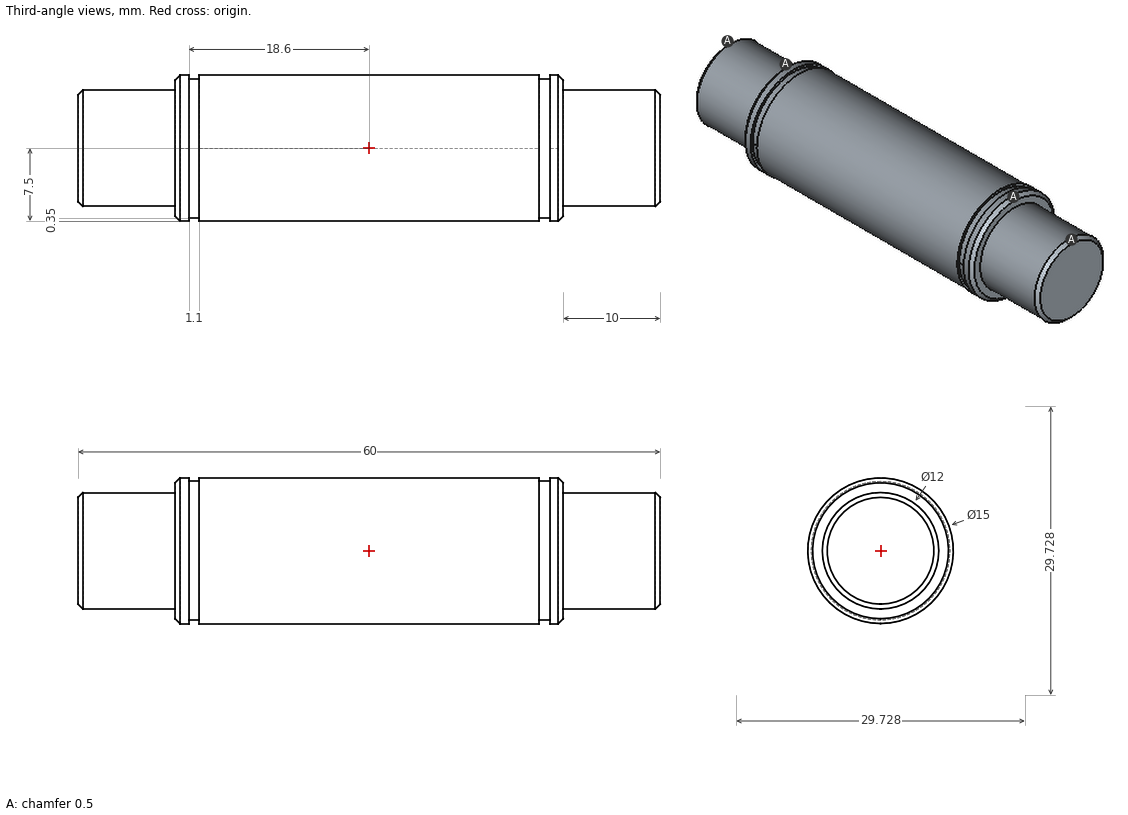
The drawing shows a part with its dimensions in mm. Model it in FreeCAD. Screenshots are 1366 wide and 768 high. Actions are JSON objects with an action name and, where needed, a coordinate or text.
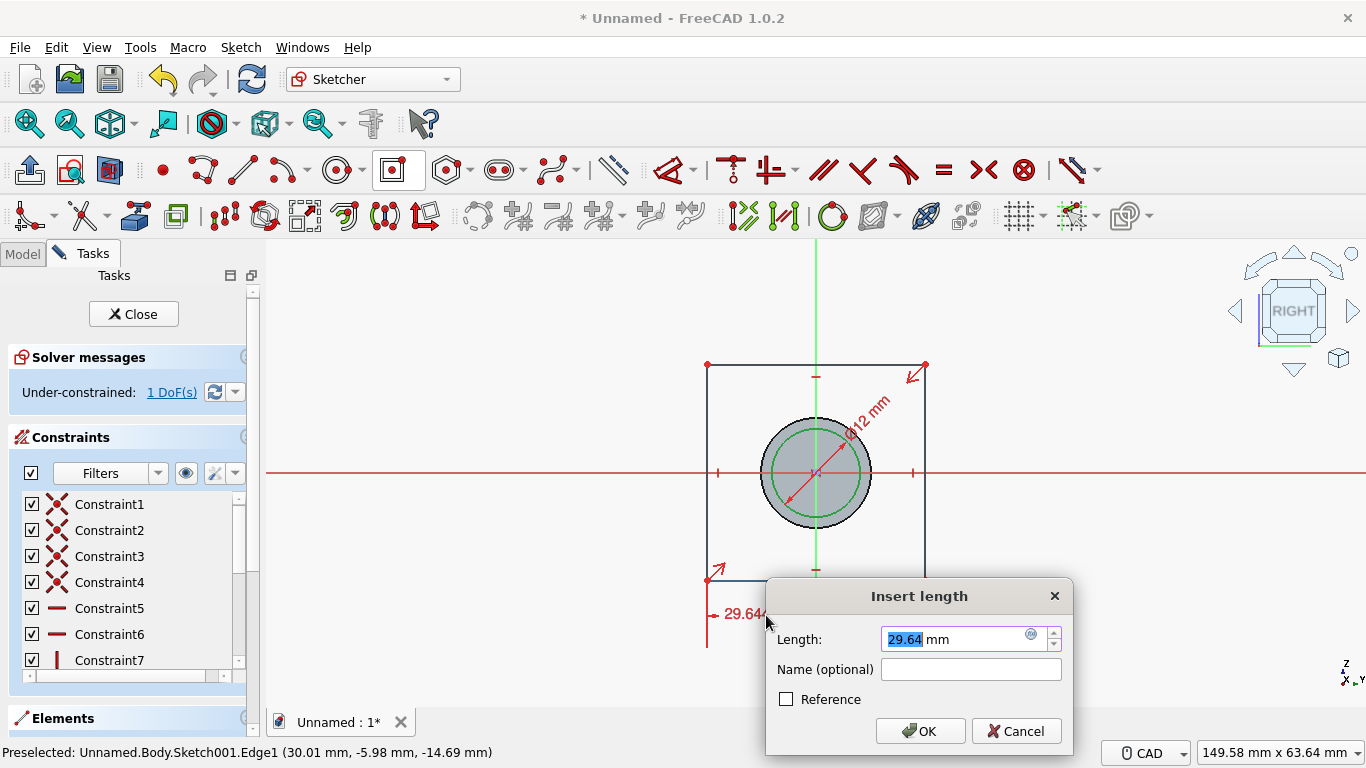
{"action": "type", "text": "29.728"}
{"action": "key", "text": "Return"}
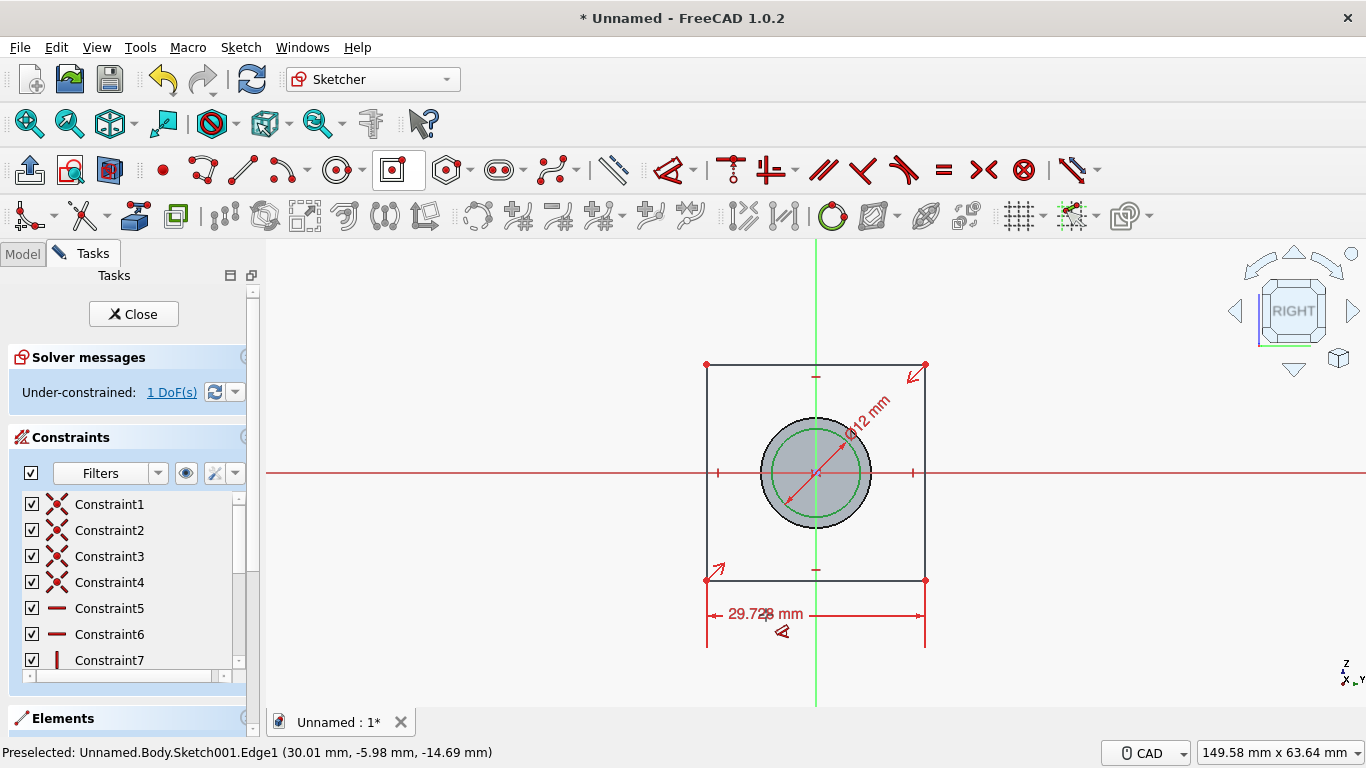
{"action": "left_click", "coordinate": [925, 516]}
{"action": "left_click", "coordinate": [959, 423]}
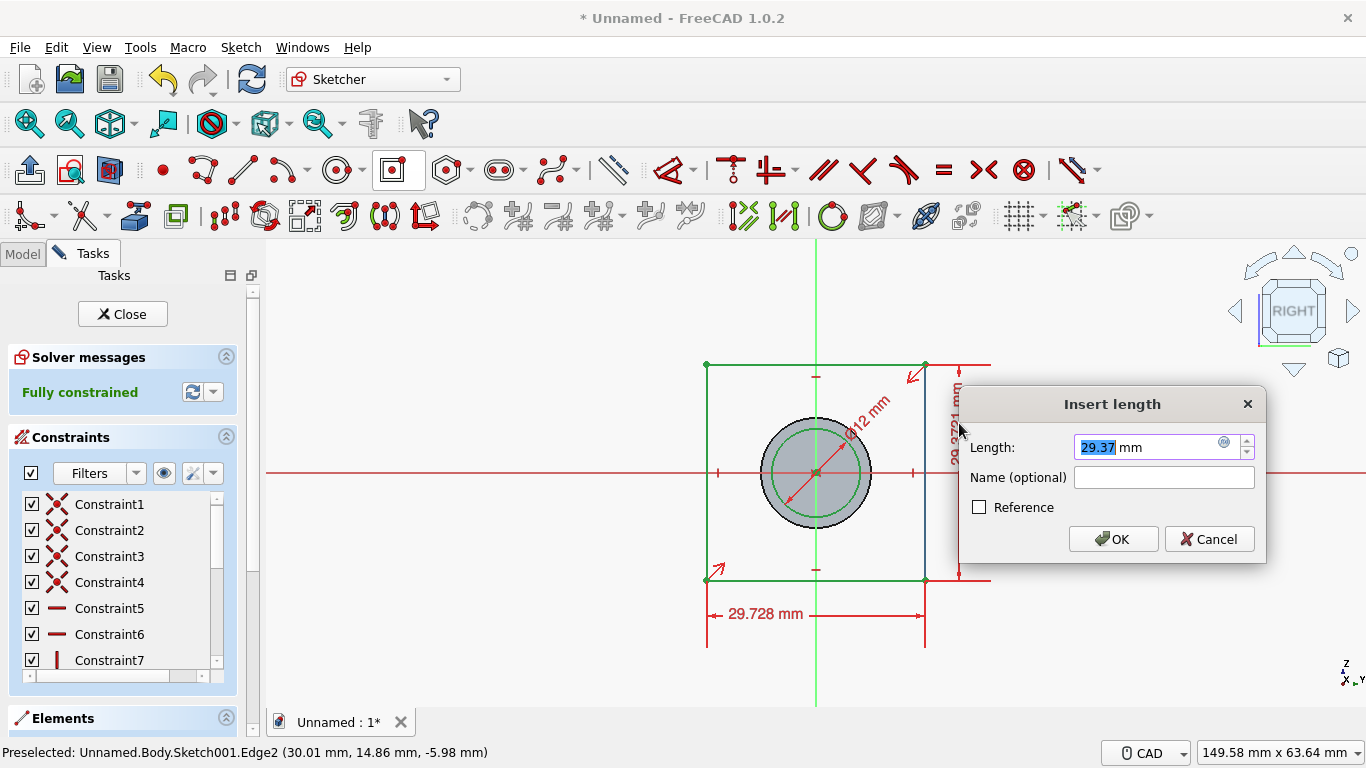
{"action": "type", "text": "29.728"}
{"action": "key", "text": "Return"}
{"action": "key", "text": "Escape"}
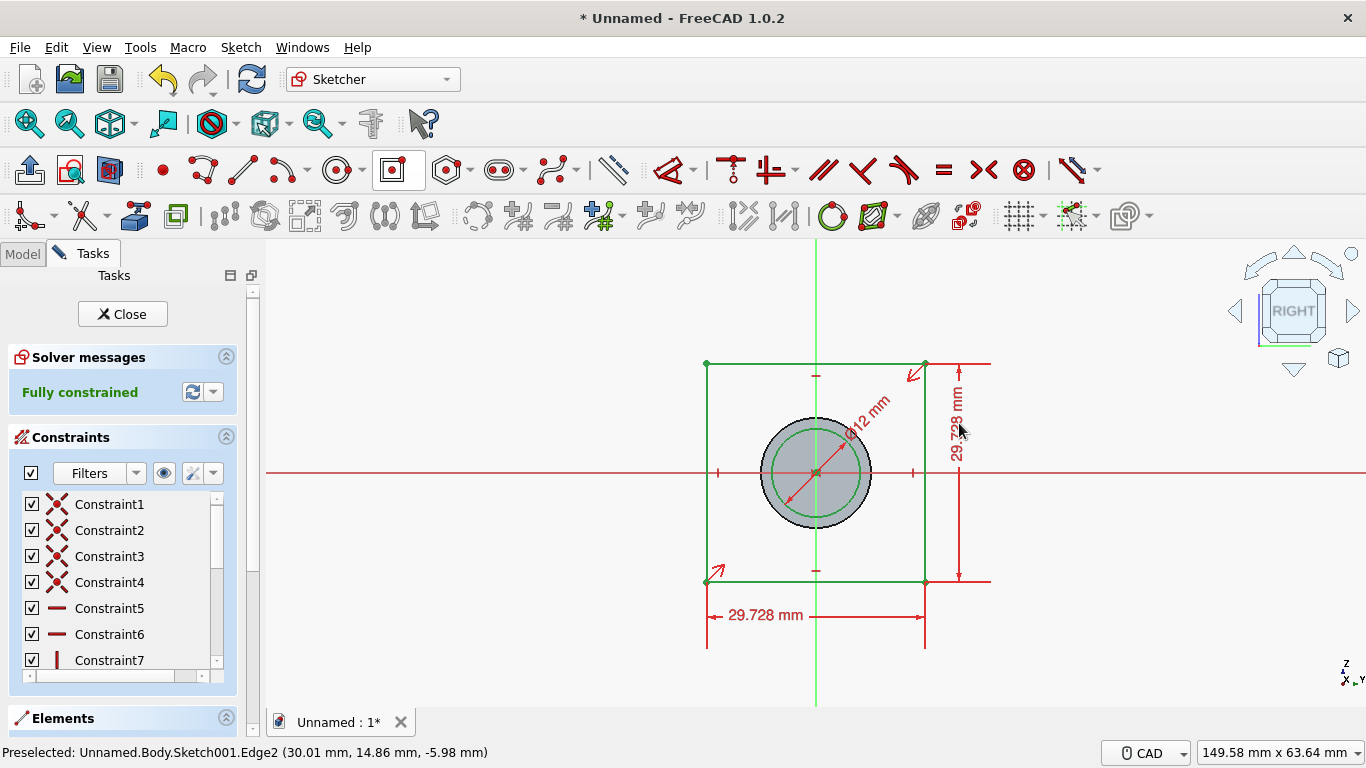
{"action": "left_click", "coordinate": [123, 314]}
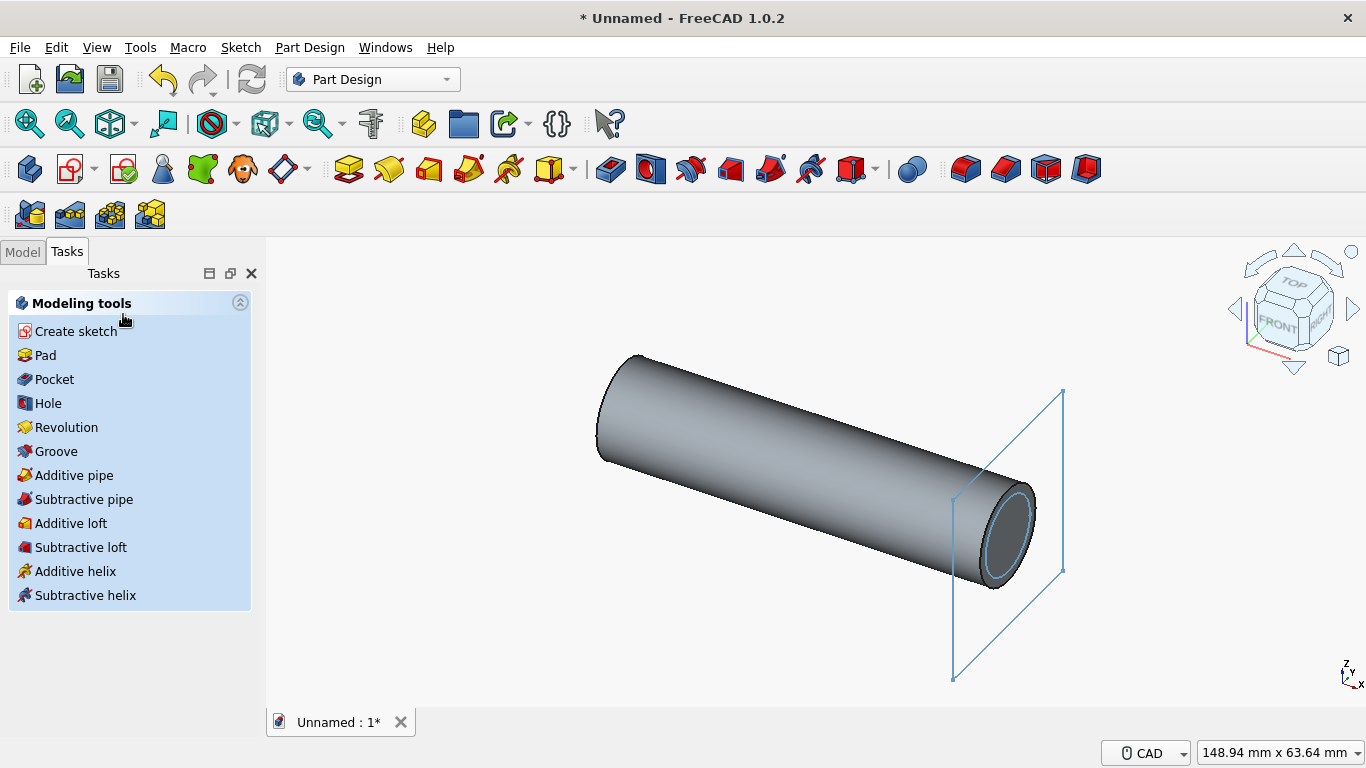
{"action": "left_click", "coordinate": [612, 170]}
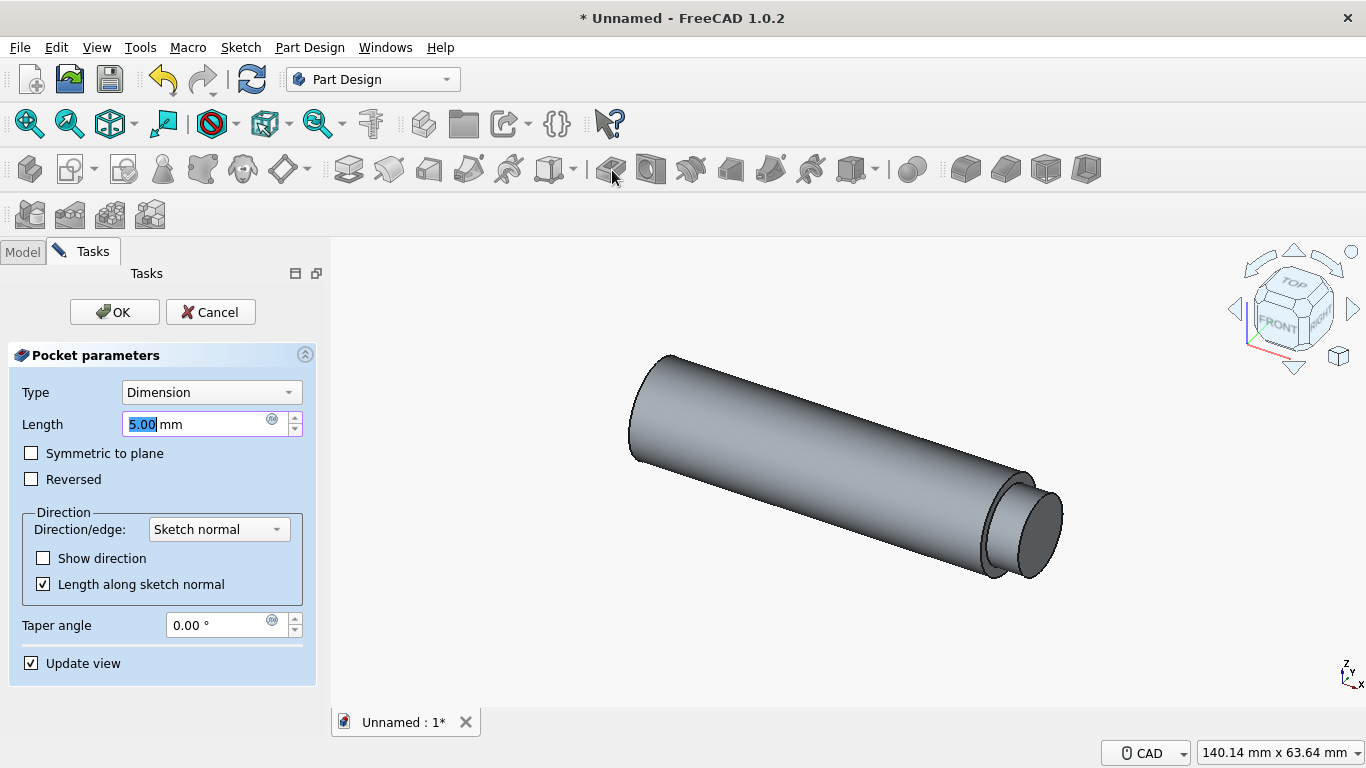
{"action": "type", "text": "10"}
{"action": "key", "text": "Tab"}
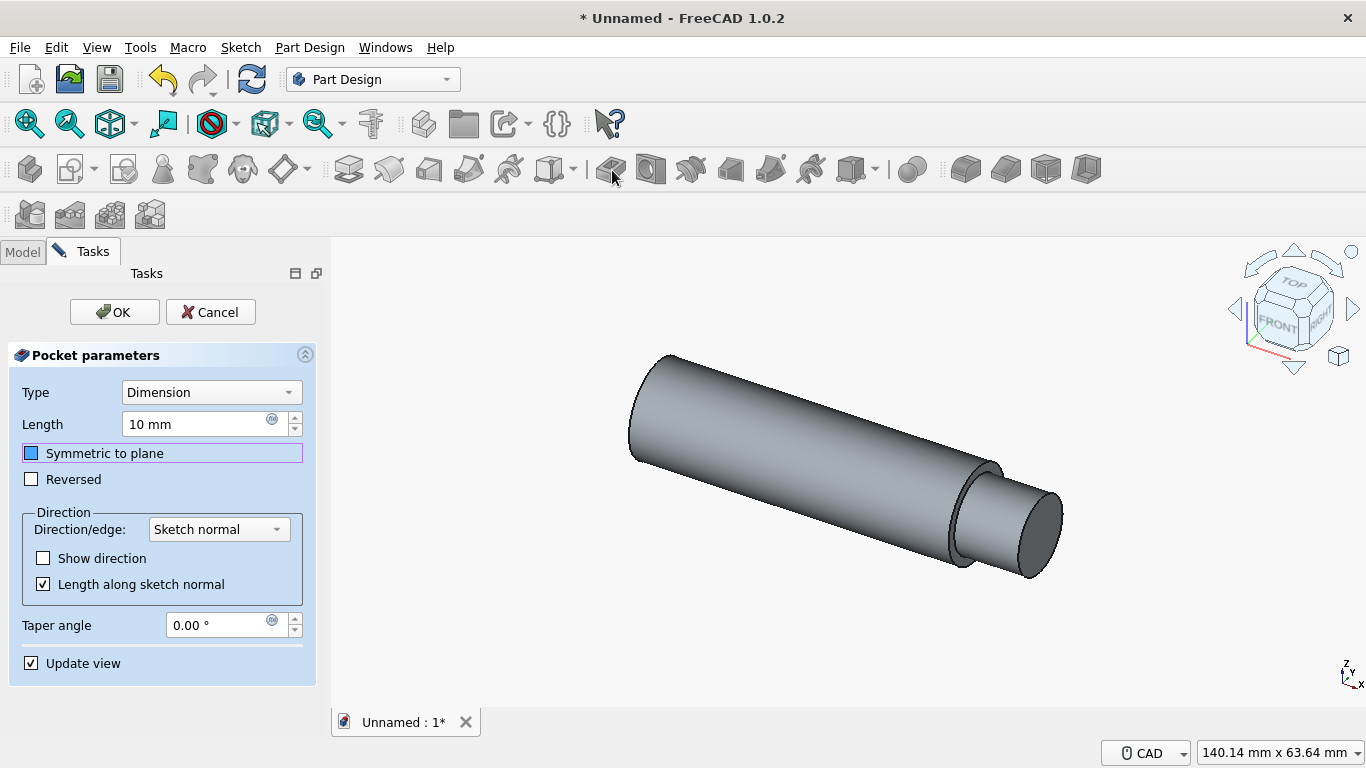
{"action": "left_click", "coordinate": [115, 312]}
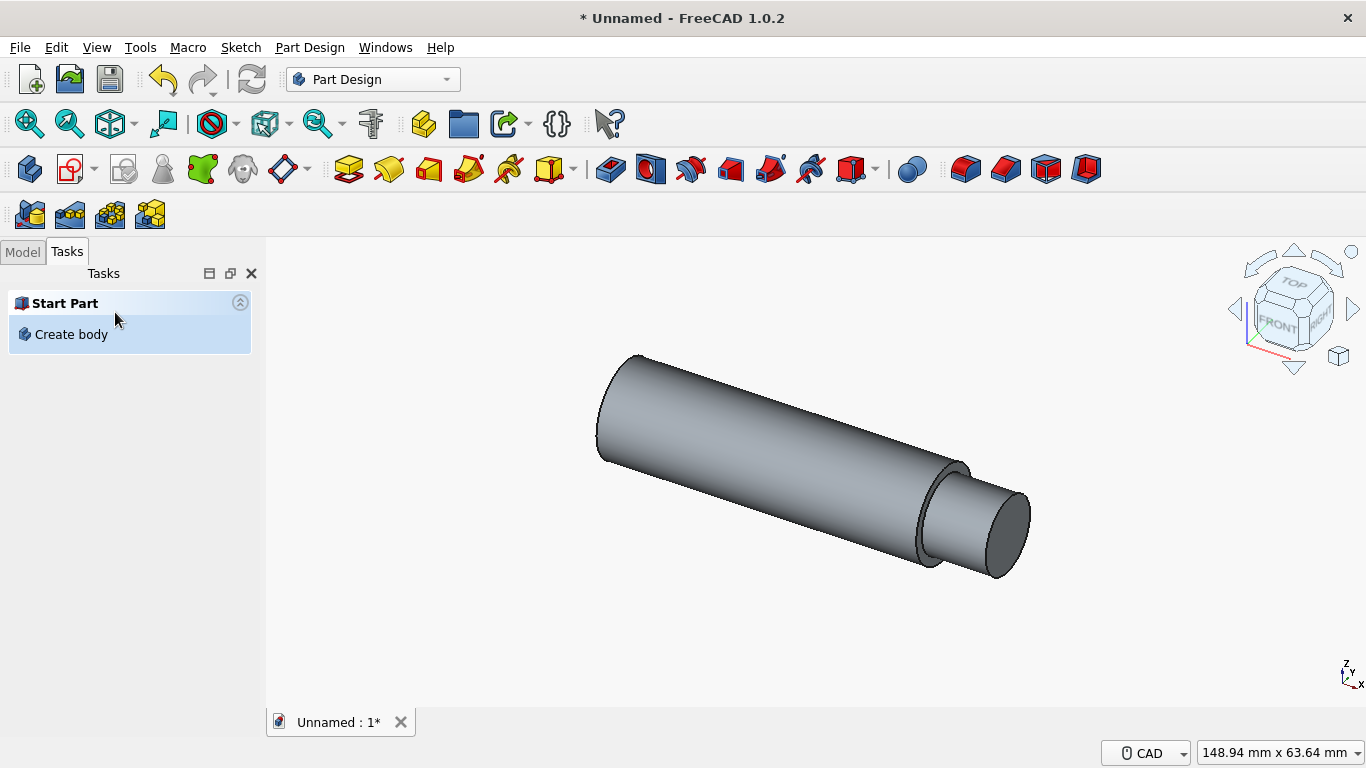
{"action": "left_click", "coordinate": [23, 251]}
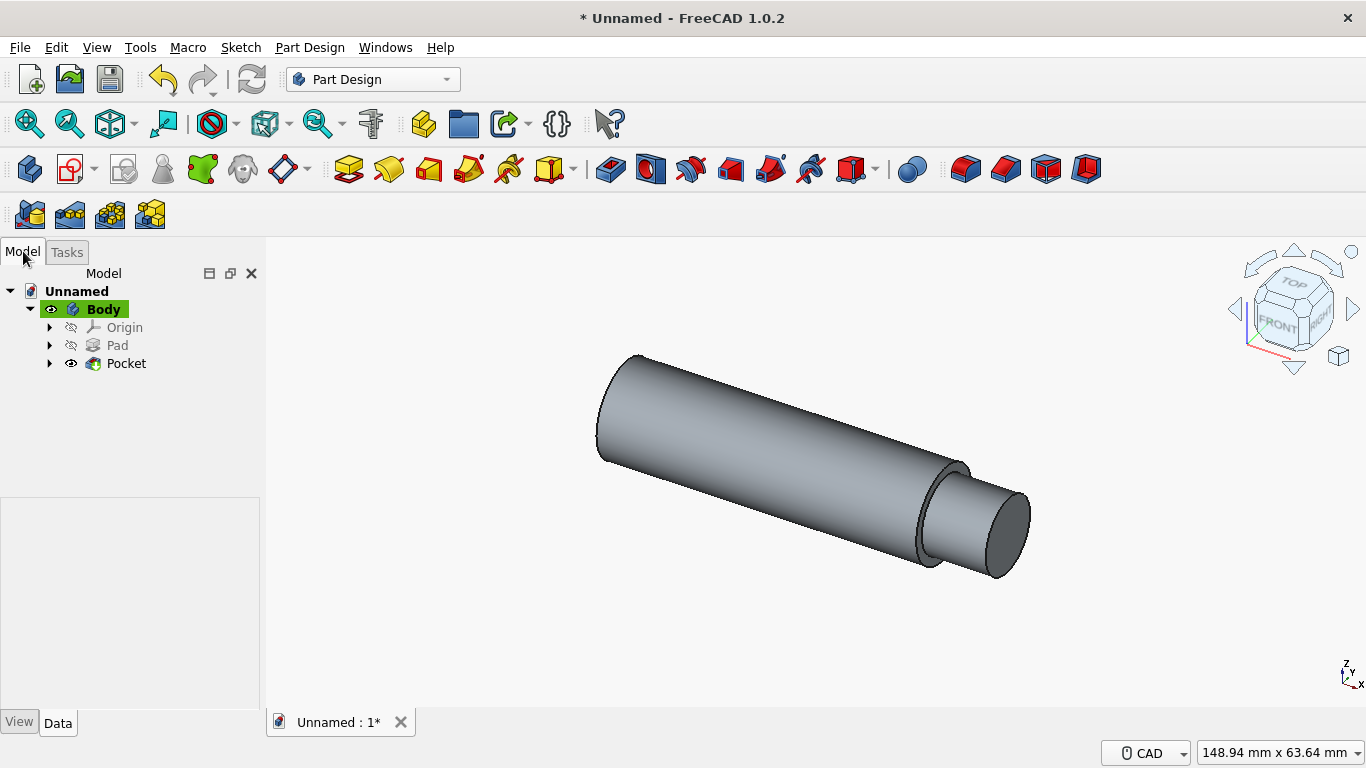
{"action": "left_click", "coordinate": [116, 363]}